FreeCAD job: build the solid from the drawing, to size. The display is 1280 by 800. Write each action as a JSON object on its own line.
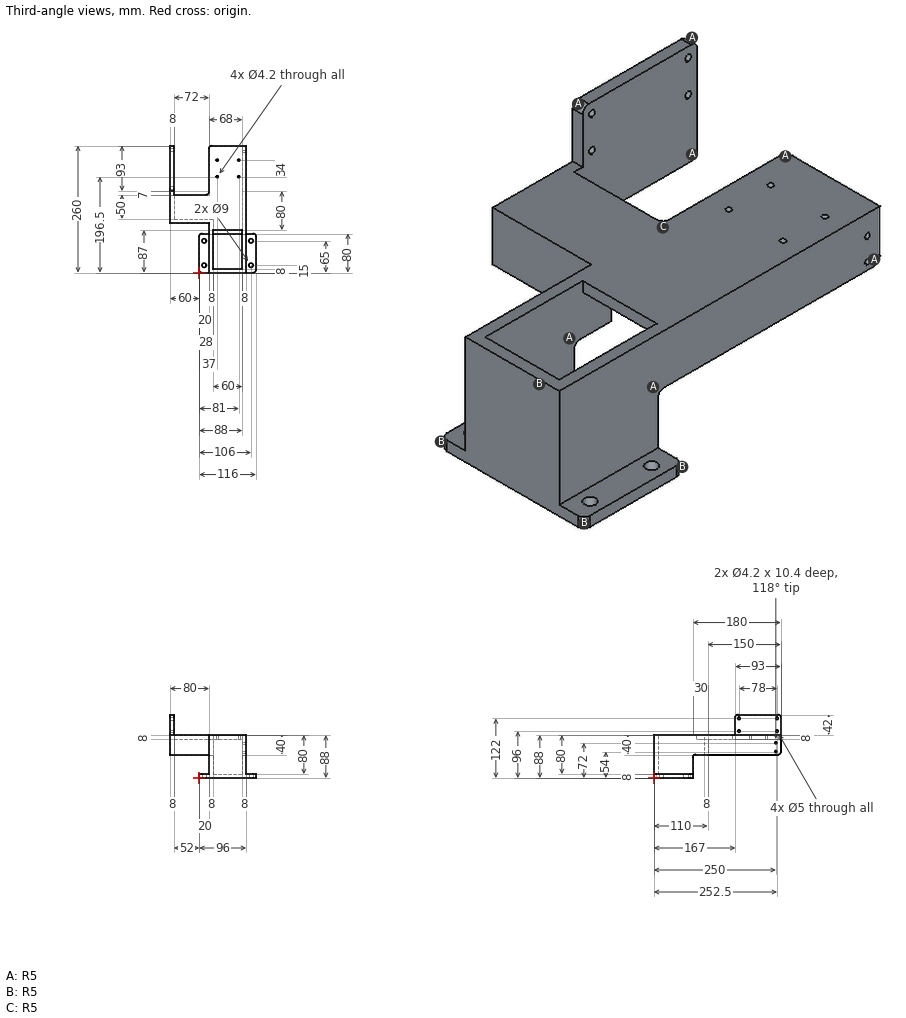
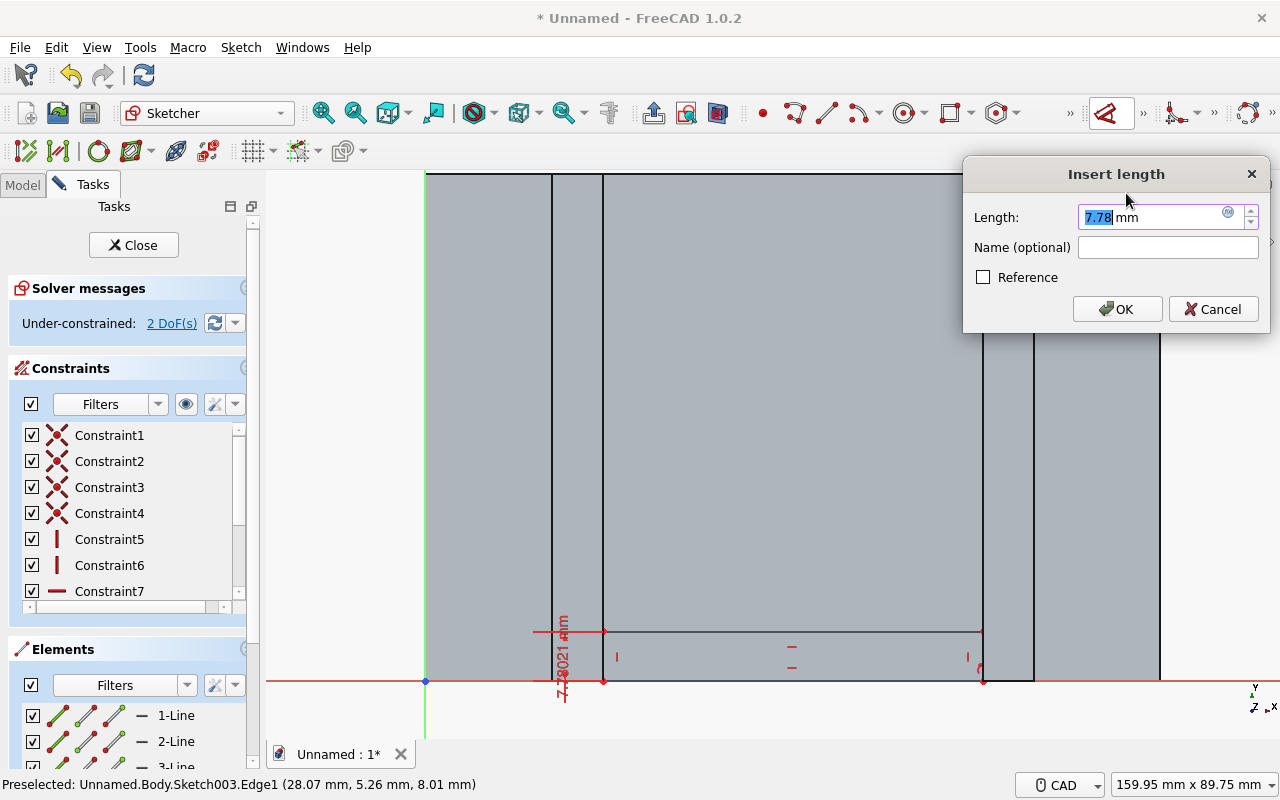
{"action": "type", "text": "8"}
{"action": "key", "text": "Return"}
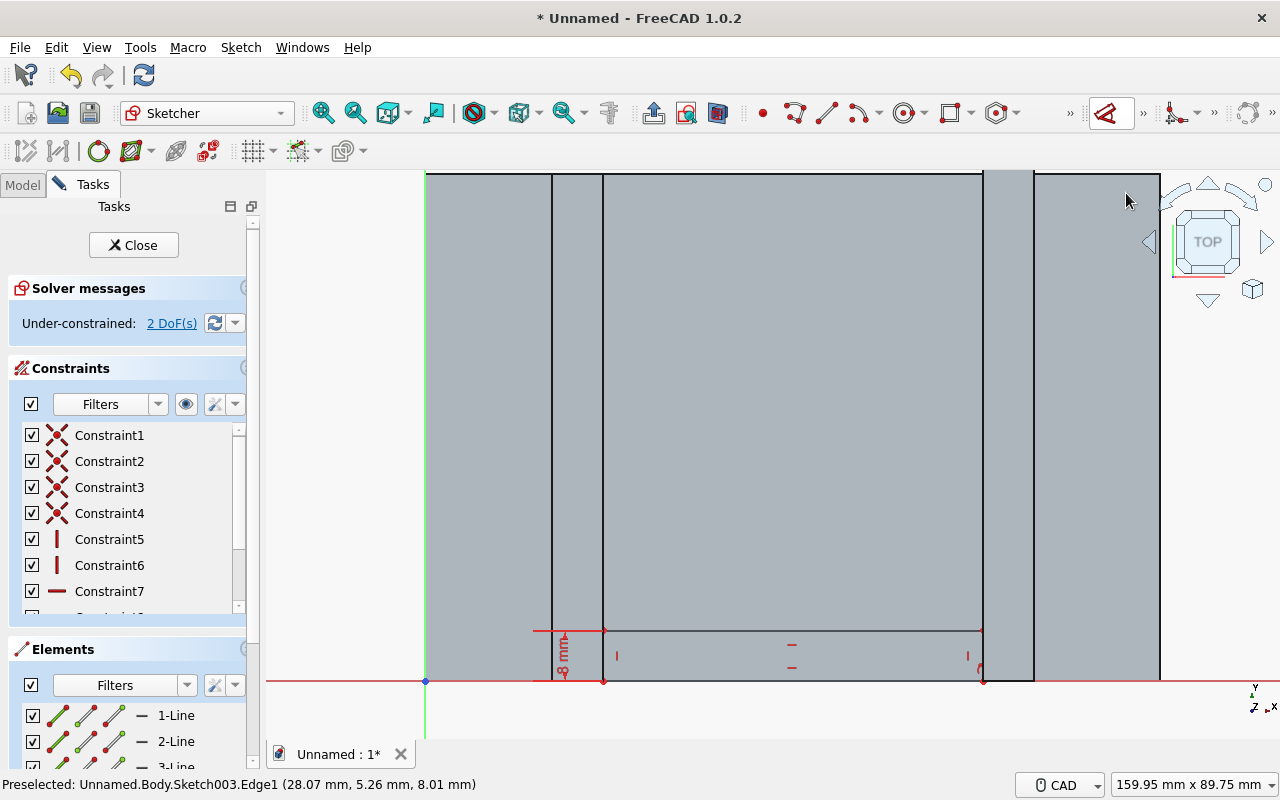
{"action": "left_click", "coordinate": [717, 681]}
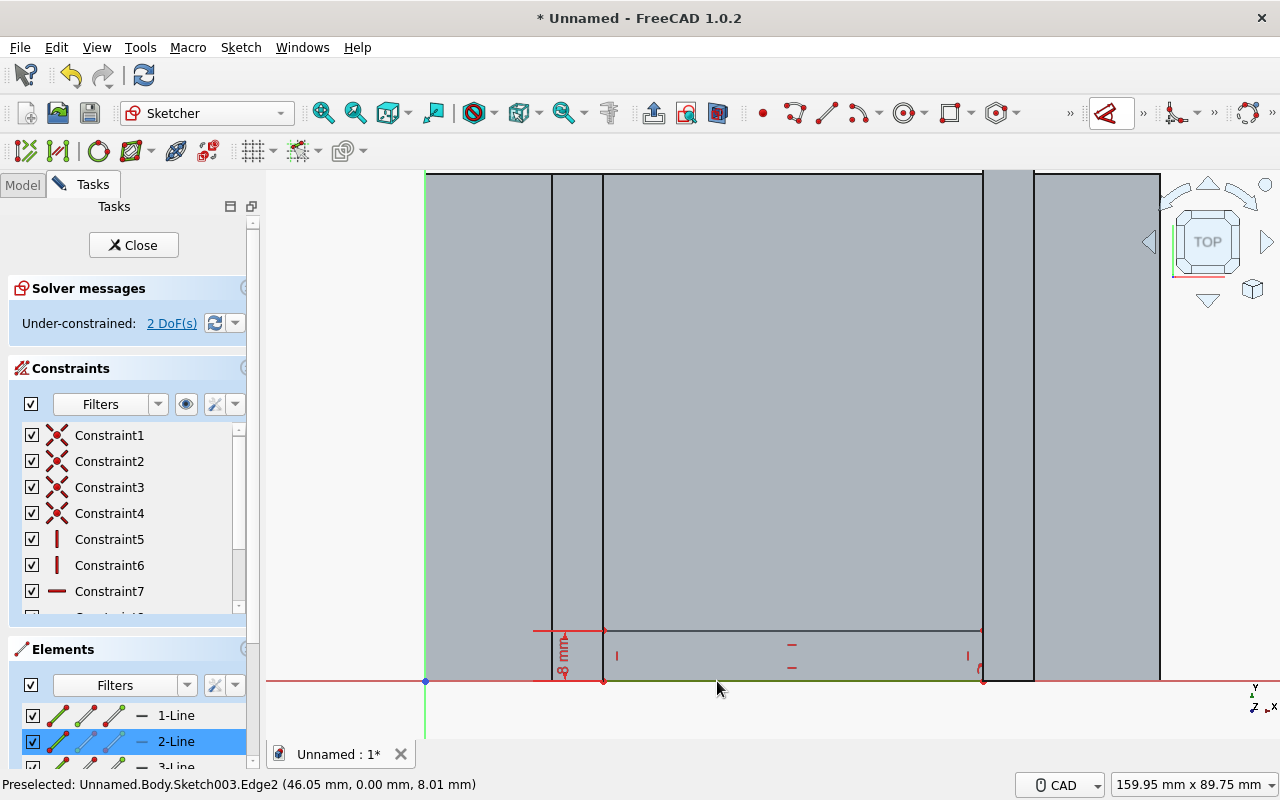
{"action": "left_click", "coordinate": [1128, 114]}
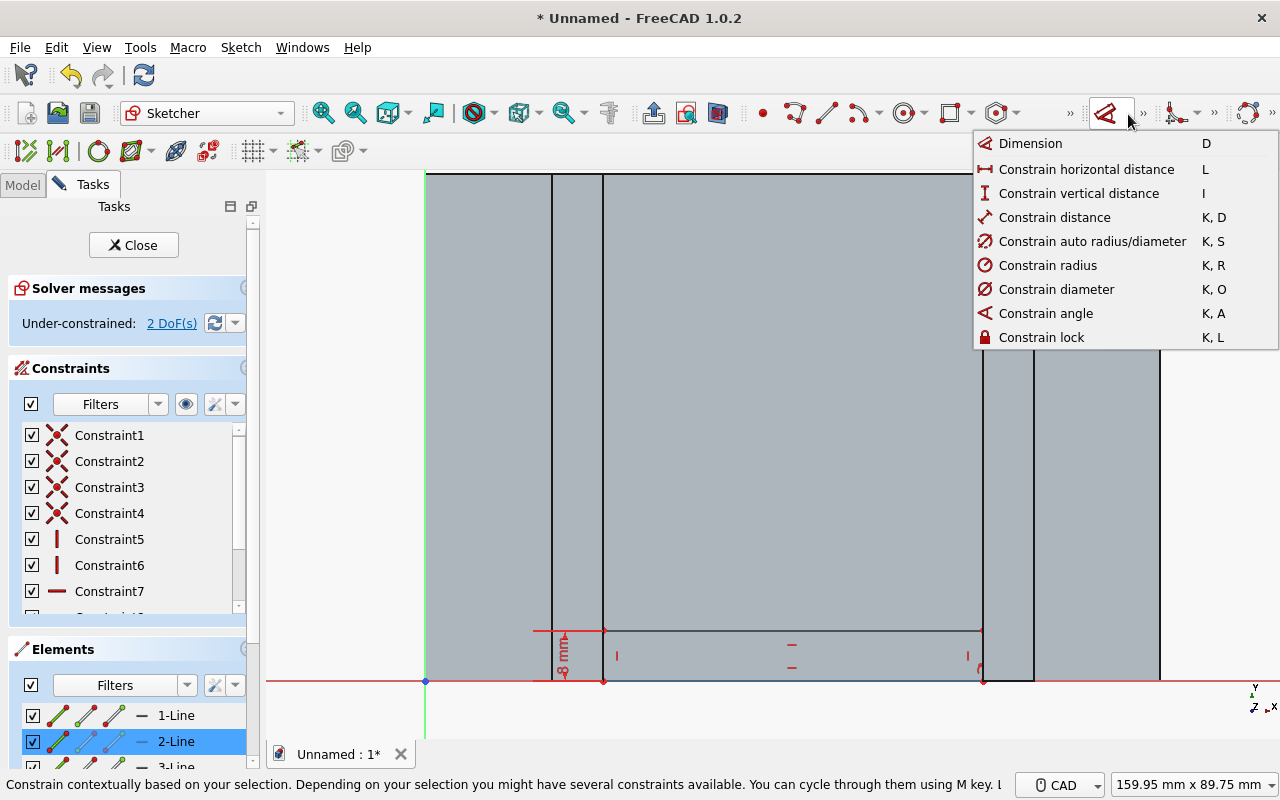
{"action": "left_click", "coordinate": [1126, 169]}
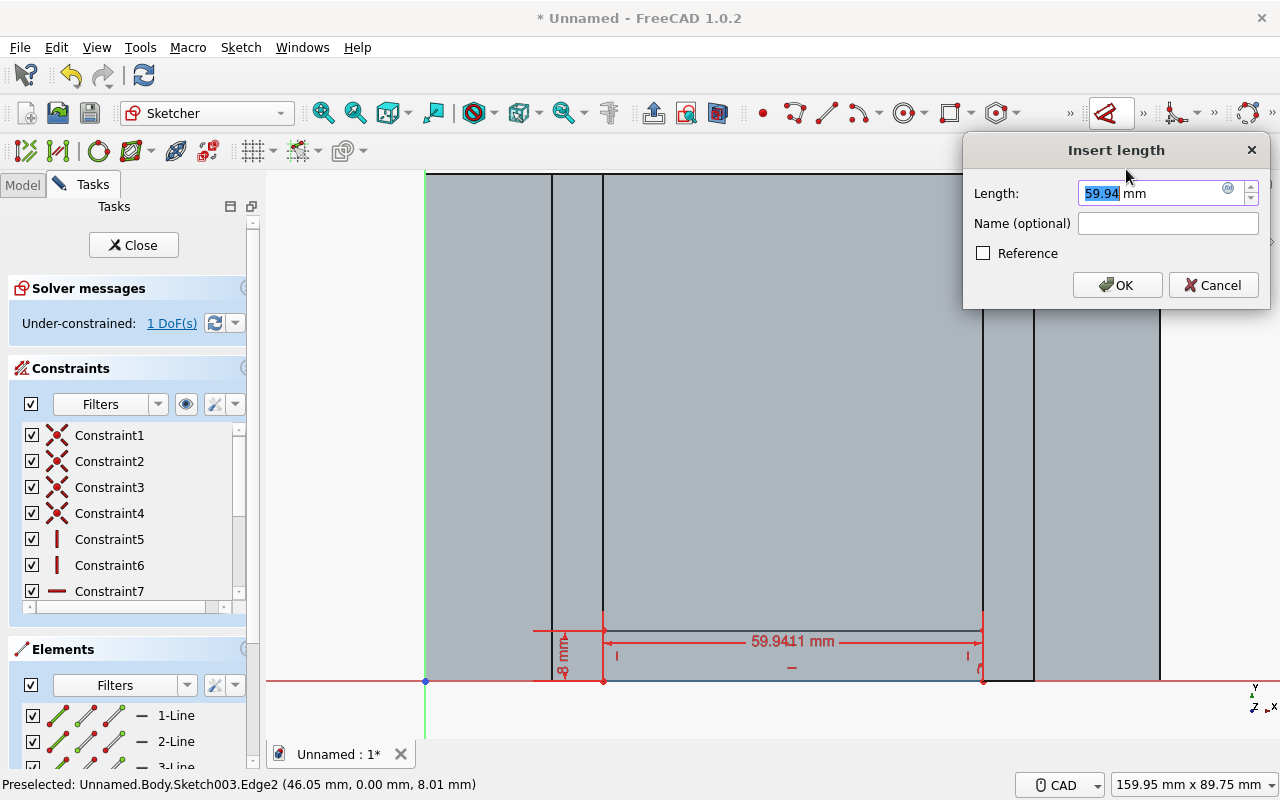
{"action": "type", "text": "60"}
{"action": "key", "text": "Return"}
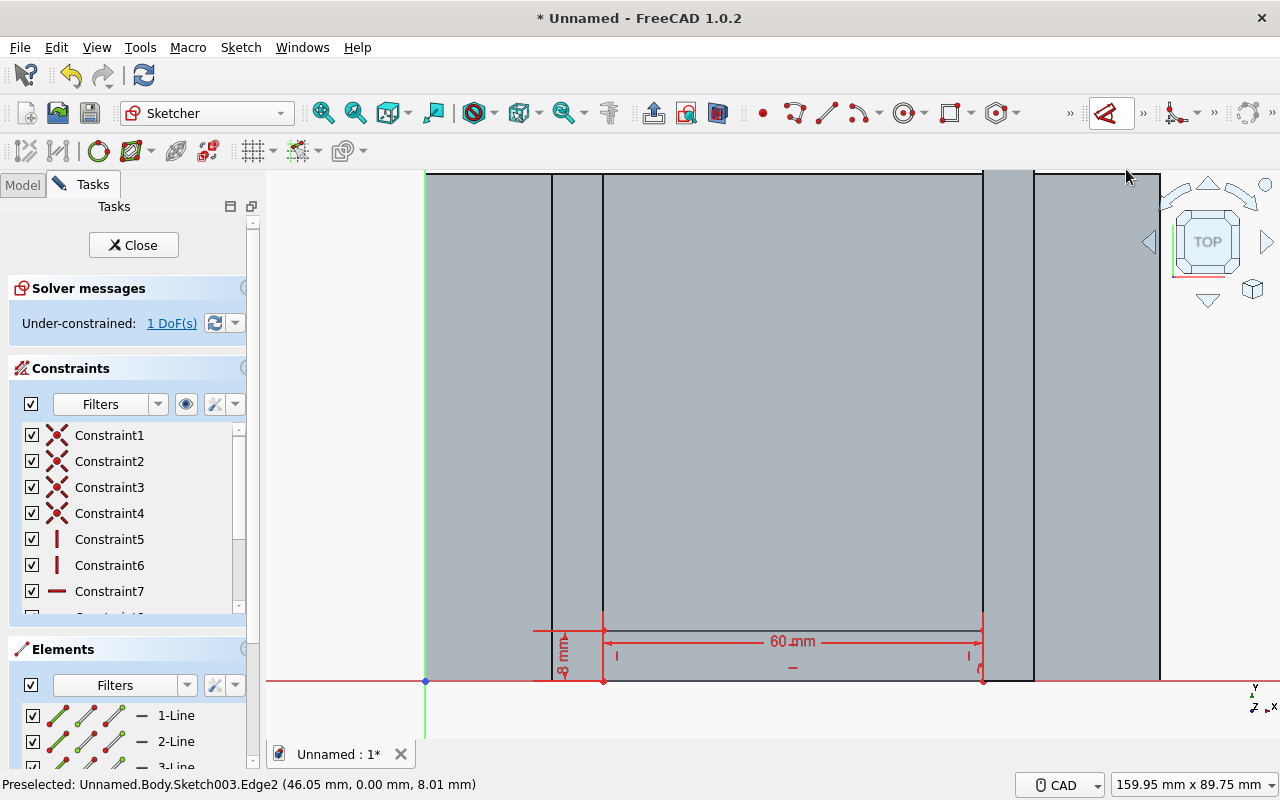
{"action": "left_click", "coordinate": [603, 631]}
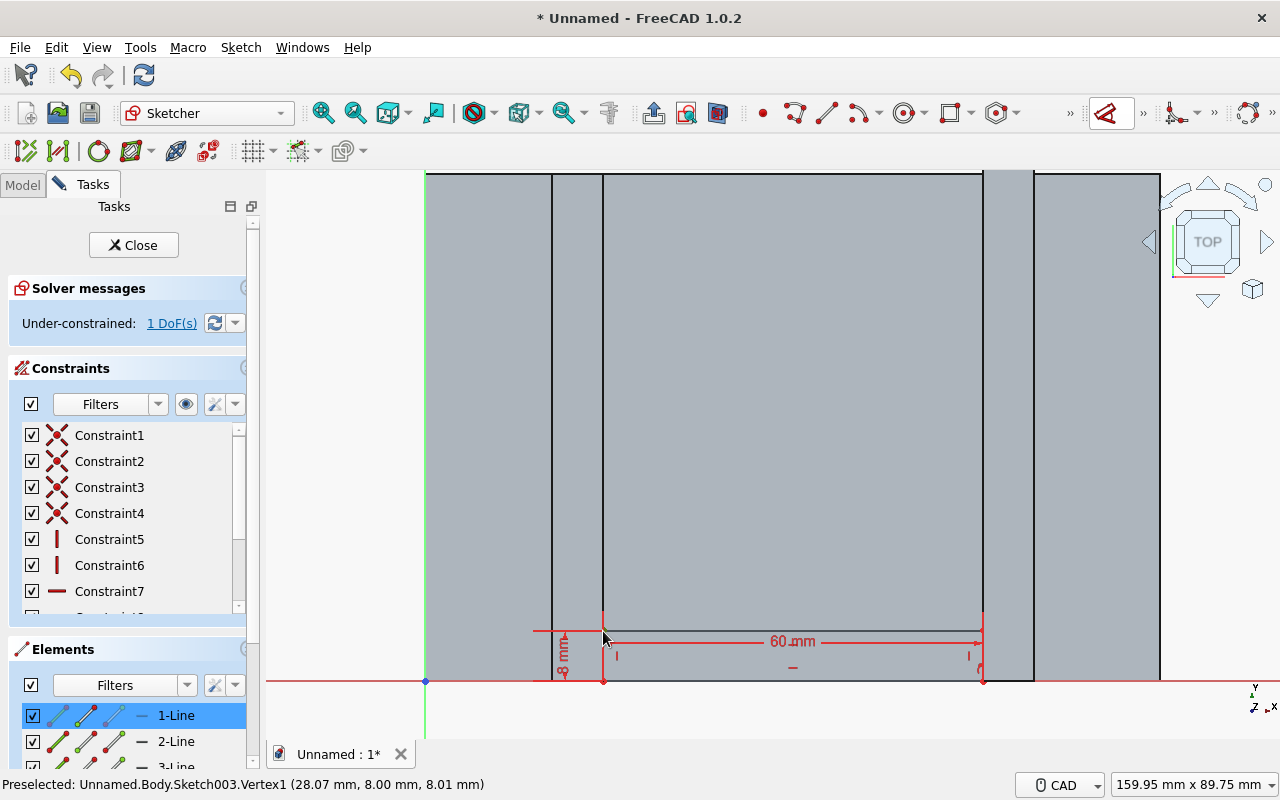
{"action": "left_click", "coordinate": [1128, 114]}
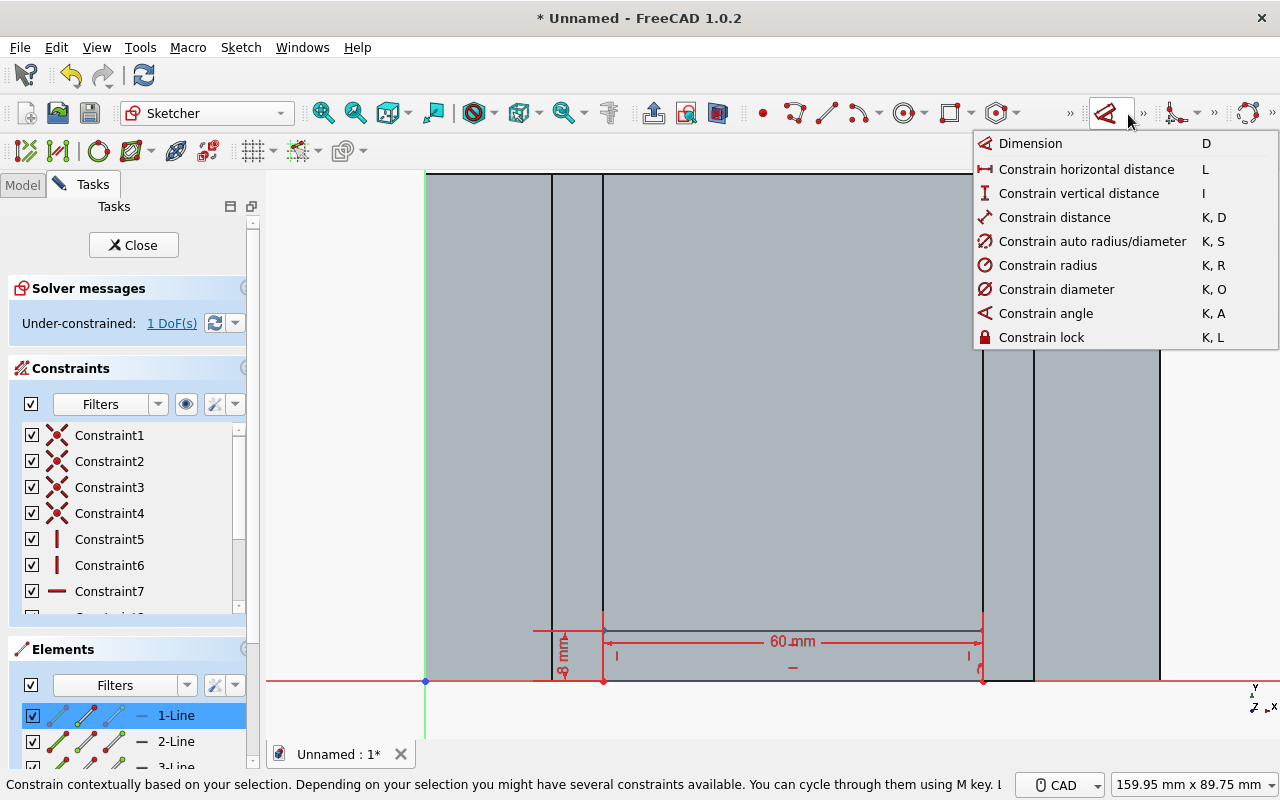
{"action": "left_click", "coordinate": [1126, 169]}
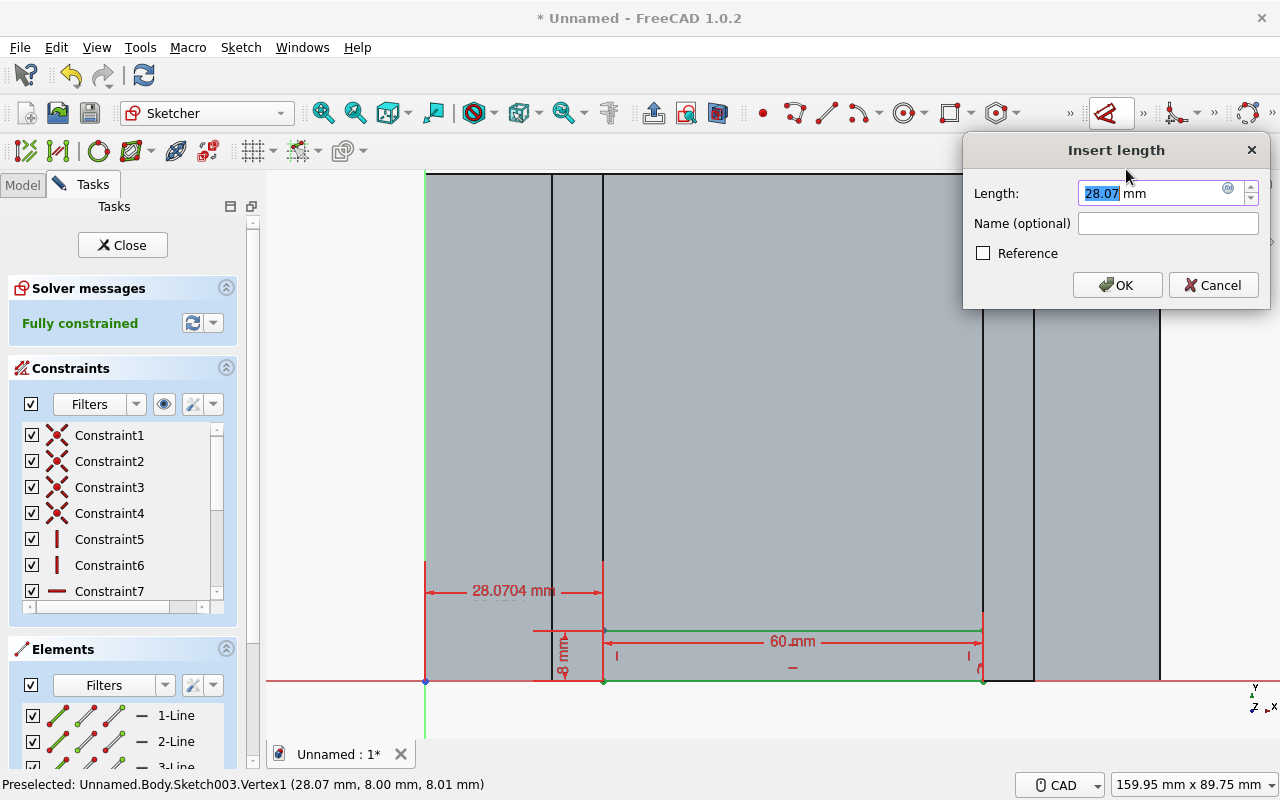
{"action": "type", "text": "28"}
{"action": "key", "text": "Return"}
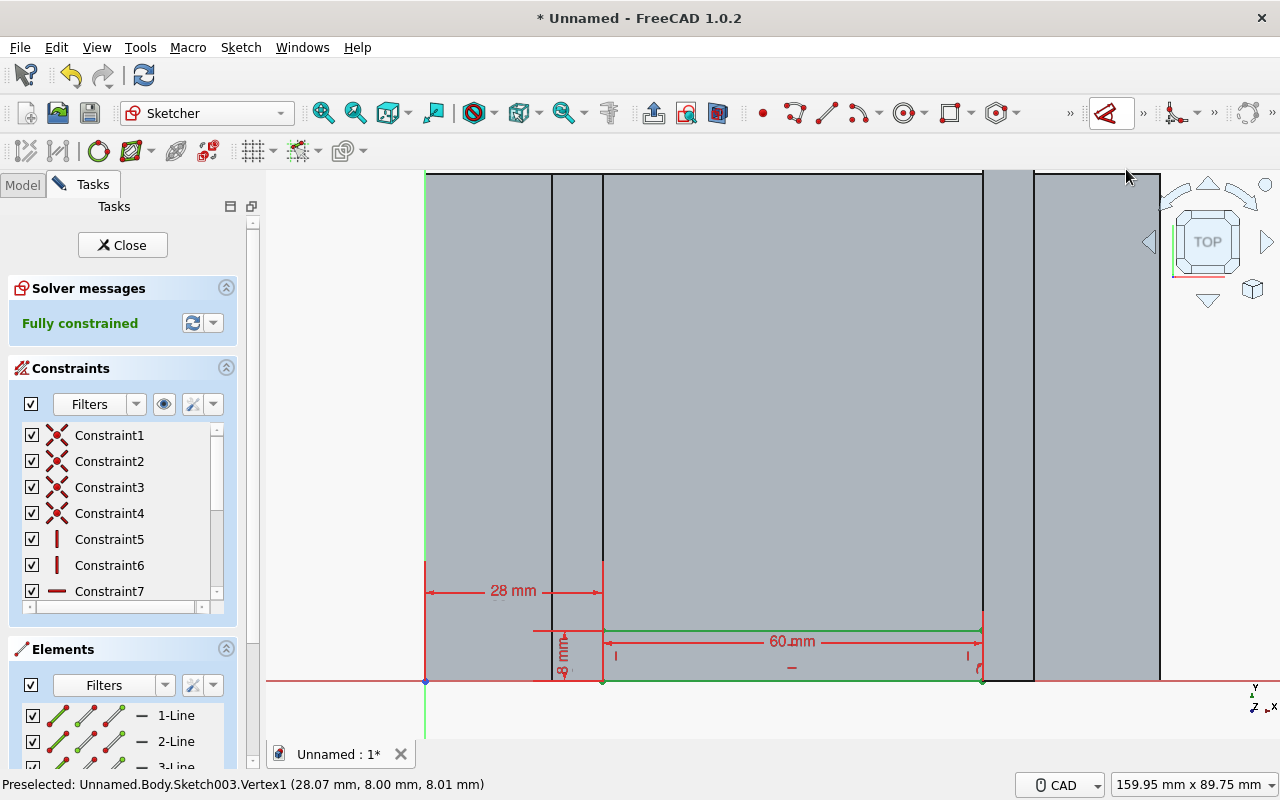
{"action": "left_click", "coordinate": [123, 245]}